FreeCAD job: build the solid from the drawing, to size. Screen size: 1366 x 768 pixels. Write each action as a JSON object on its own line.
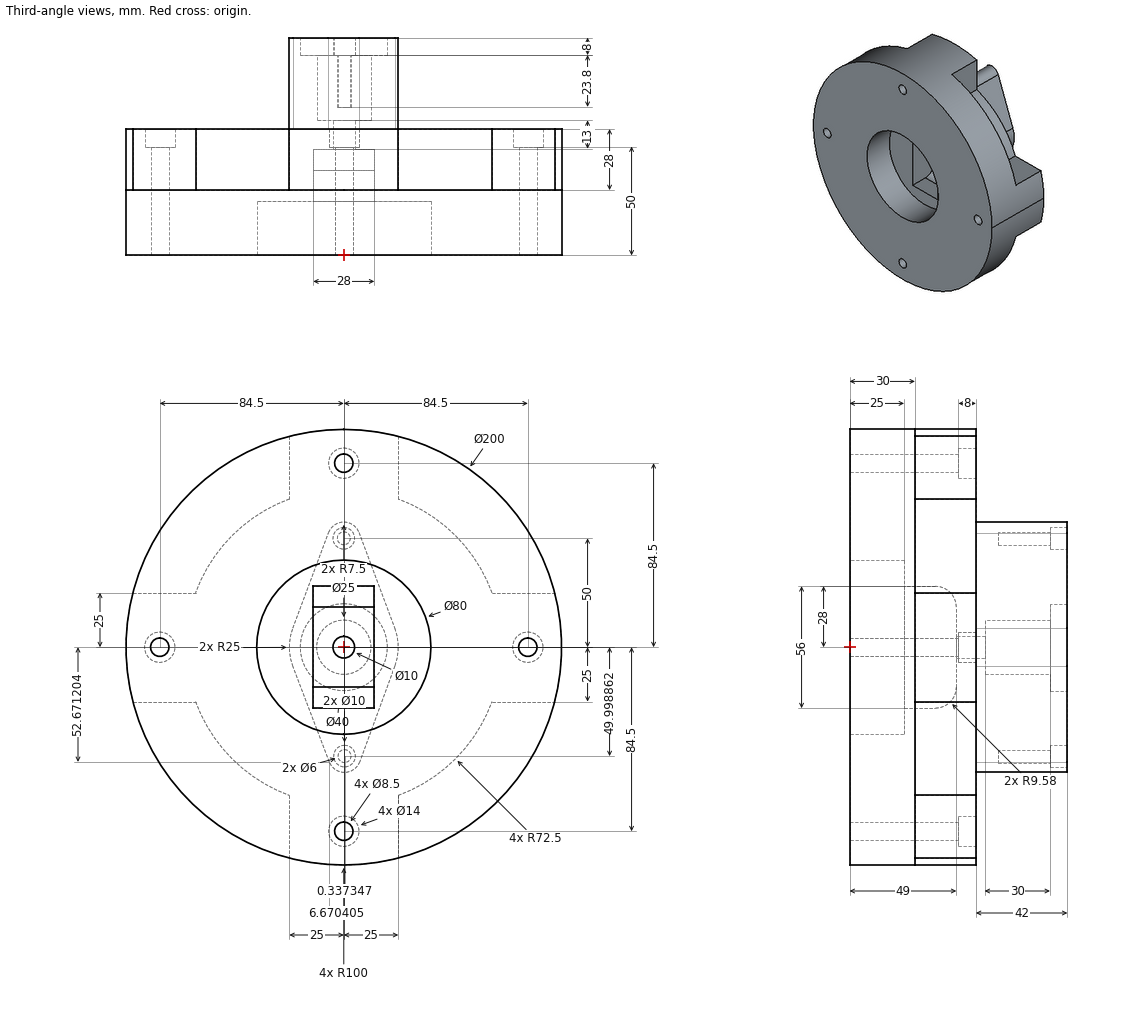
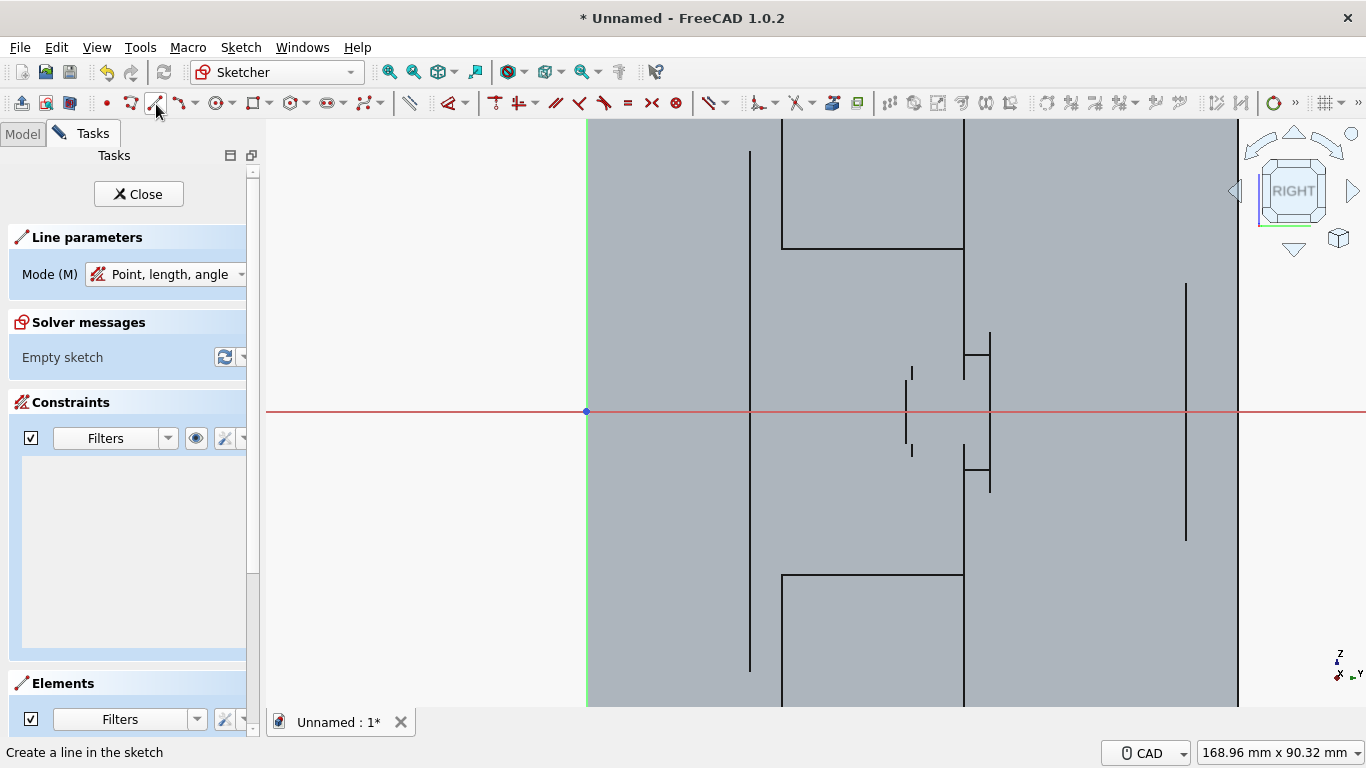
{"action": "left_click", "coordinate": [906, 532]}
{"action": "left_click", "coordinate": [906, 292]}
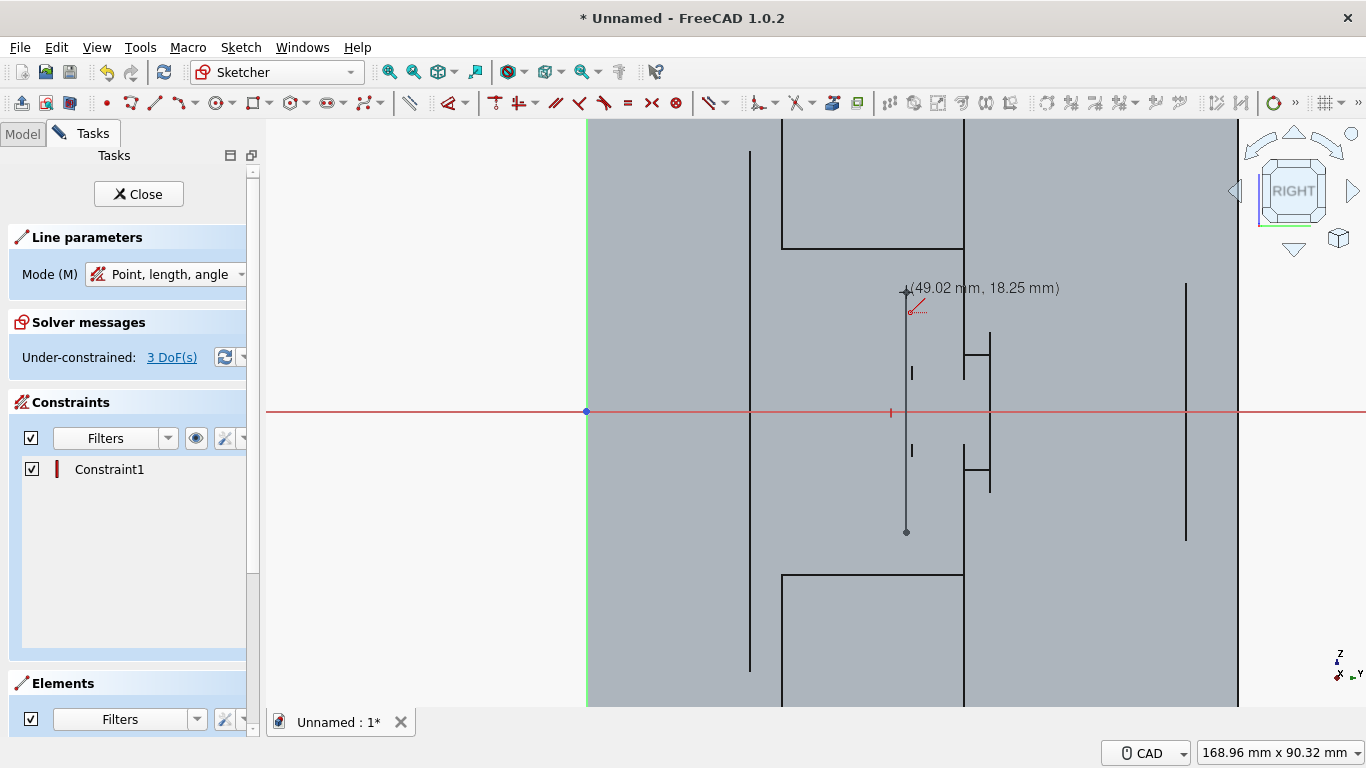
{"action": "key", "text": "g m"}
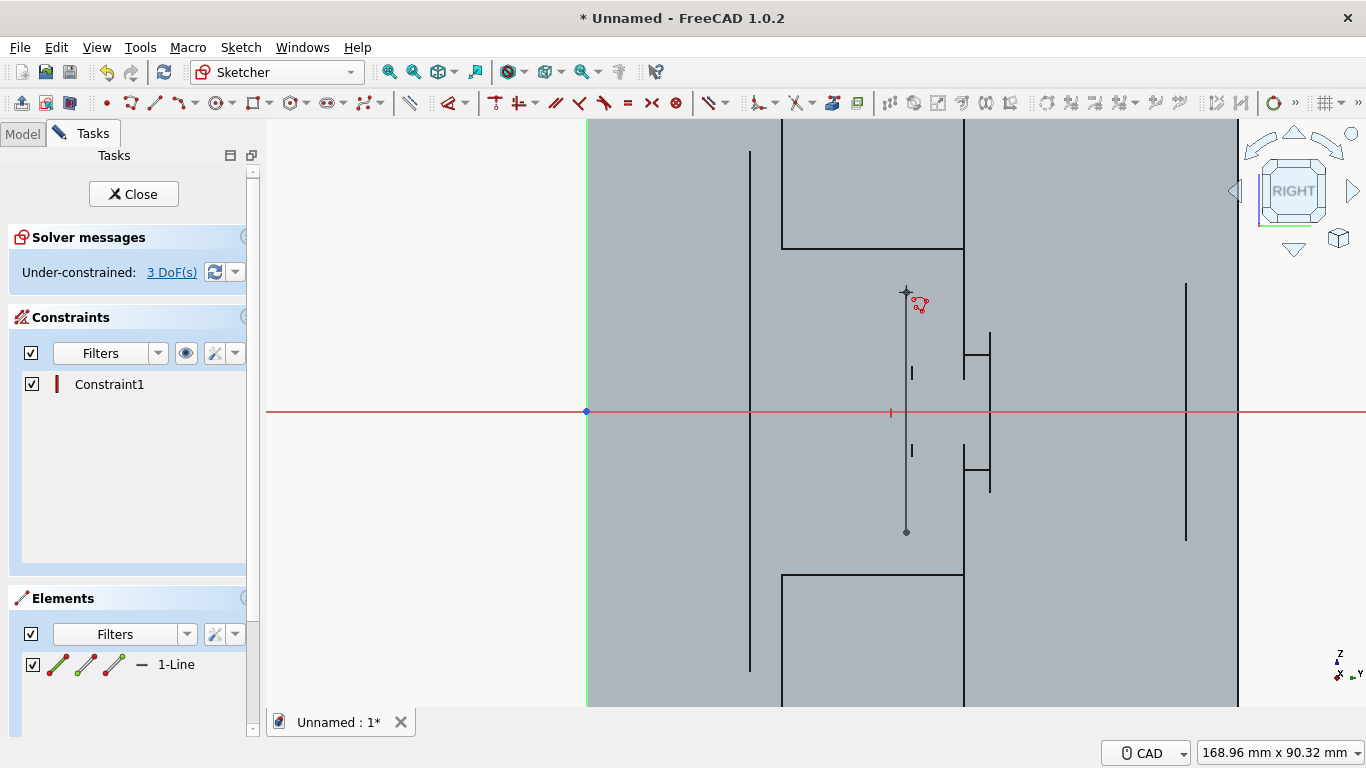
{"action": "left_click", "coordinate": [843, 230]}
{"action": "left_click", "coordinate": [750, 230]}
{"action": "left_click", "coordinate": [750, 594]}
{"action": "left_click", "coordinate": [843, 594]}
{"action": "right_click", "coordinate": [843, 594]}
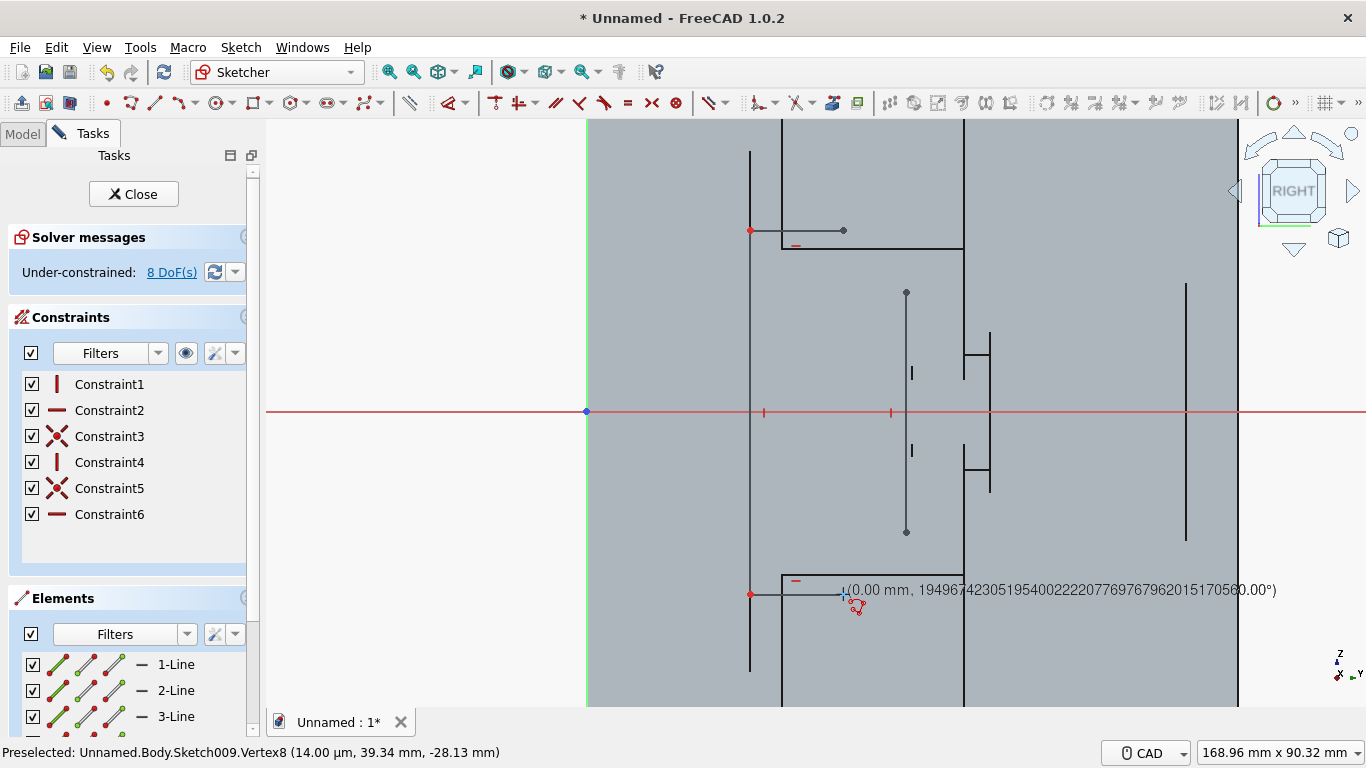
{"action": "key", "text": "g 3 a"}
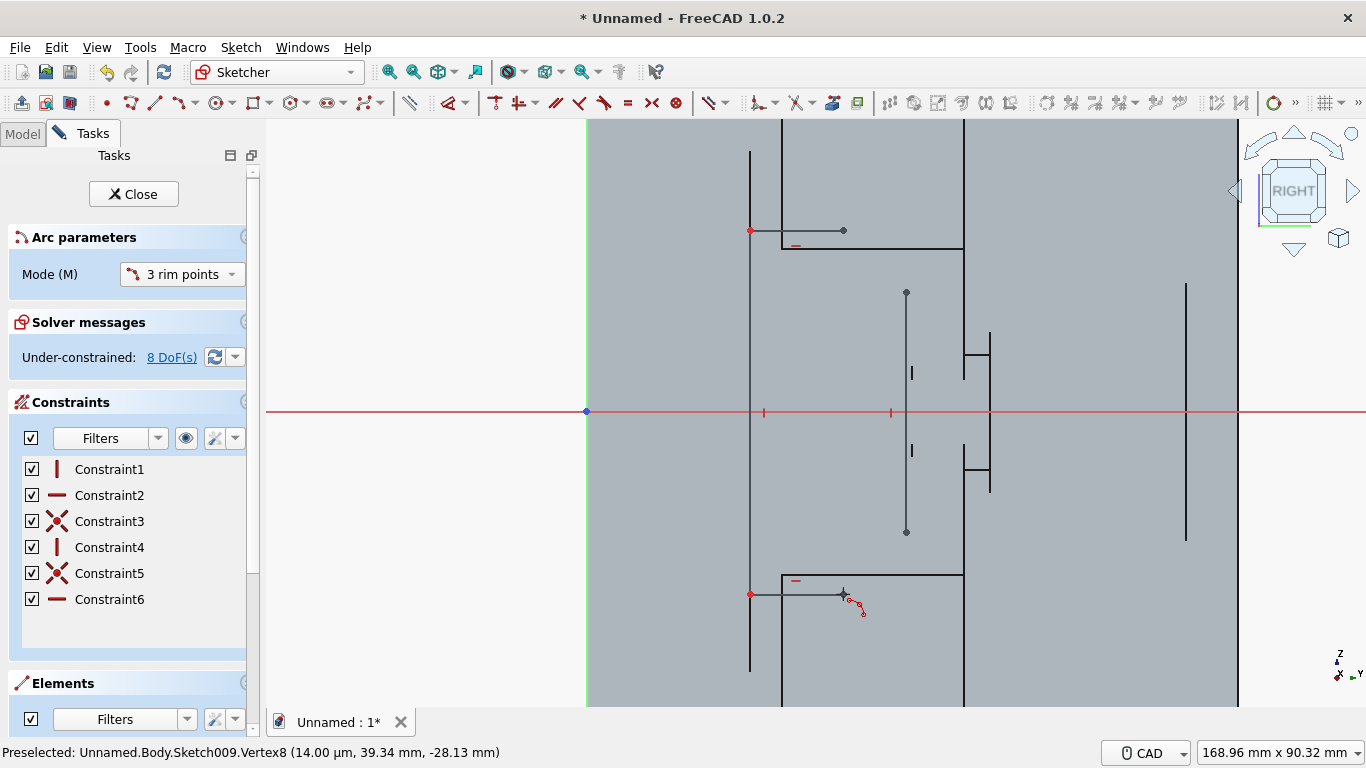
{"action": "left_click", "coordinate": [906, 293]}
{"action": "left_click", "coordinate": [843, 231]}
{"action": "left_click", "coordinate": [888, 248]}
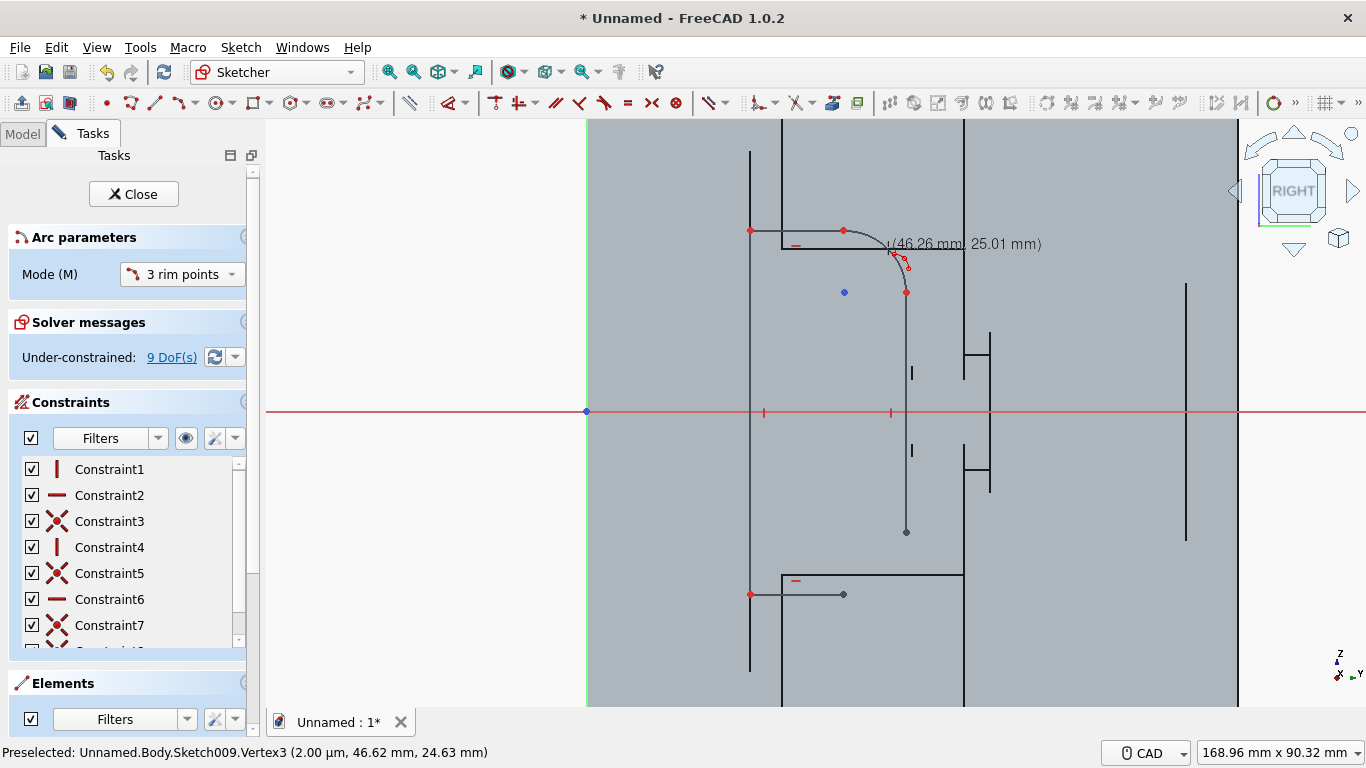
{"action": "left_click", "coordinate": [843, 595]}
{"action": "left_click", "coordinate": [906, 533]}
{"action": "left_click", "coordinate": [888, 576]}
{"action": "key", "text": "Escape"}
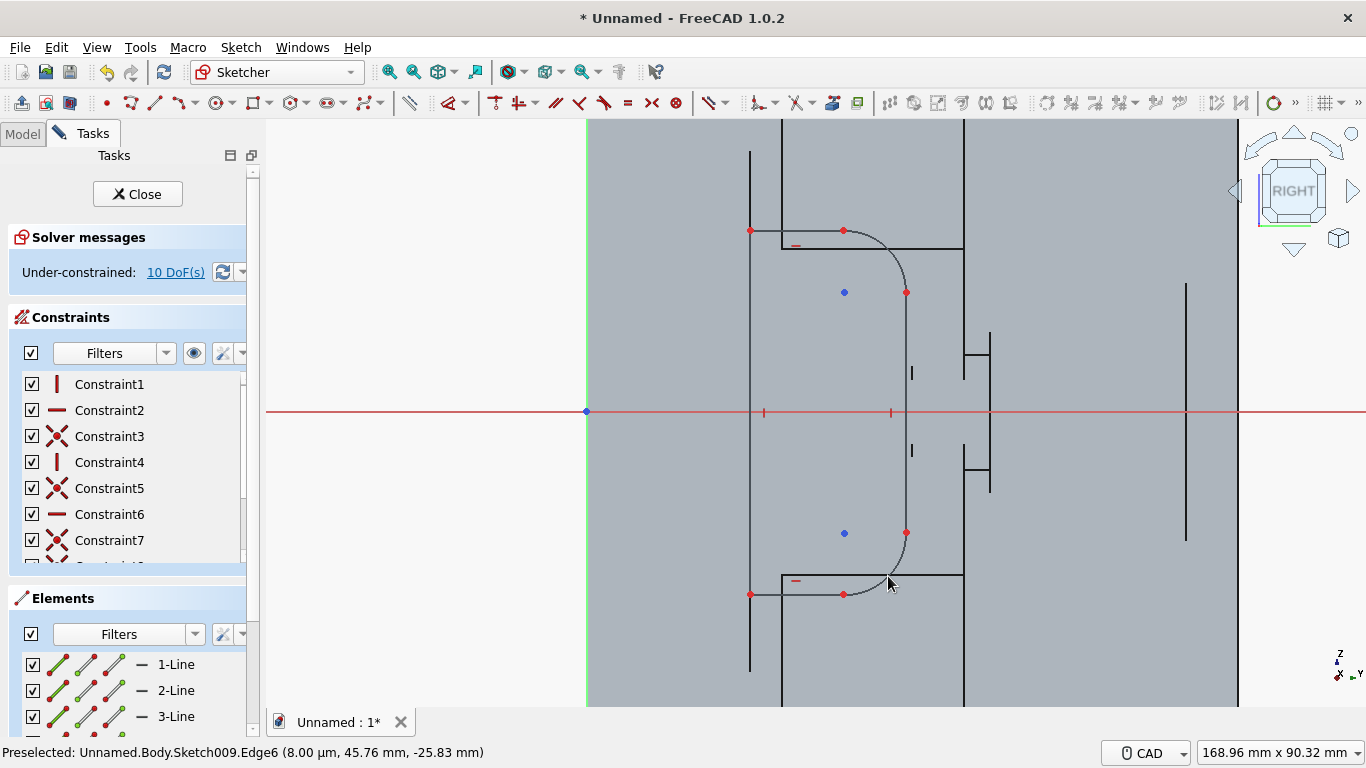
{"action": "left_click", "coordinate": [906, 461]}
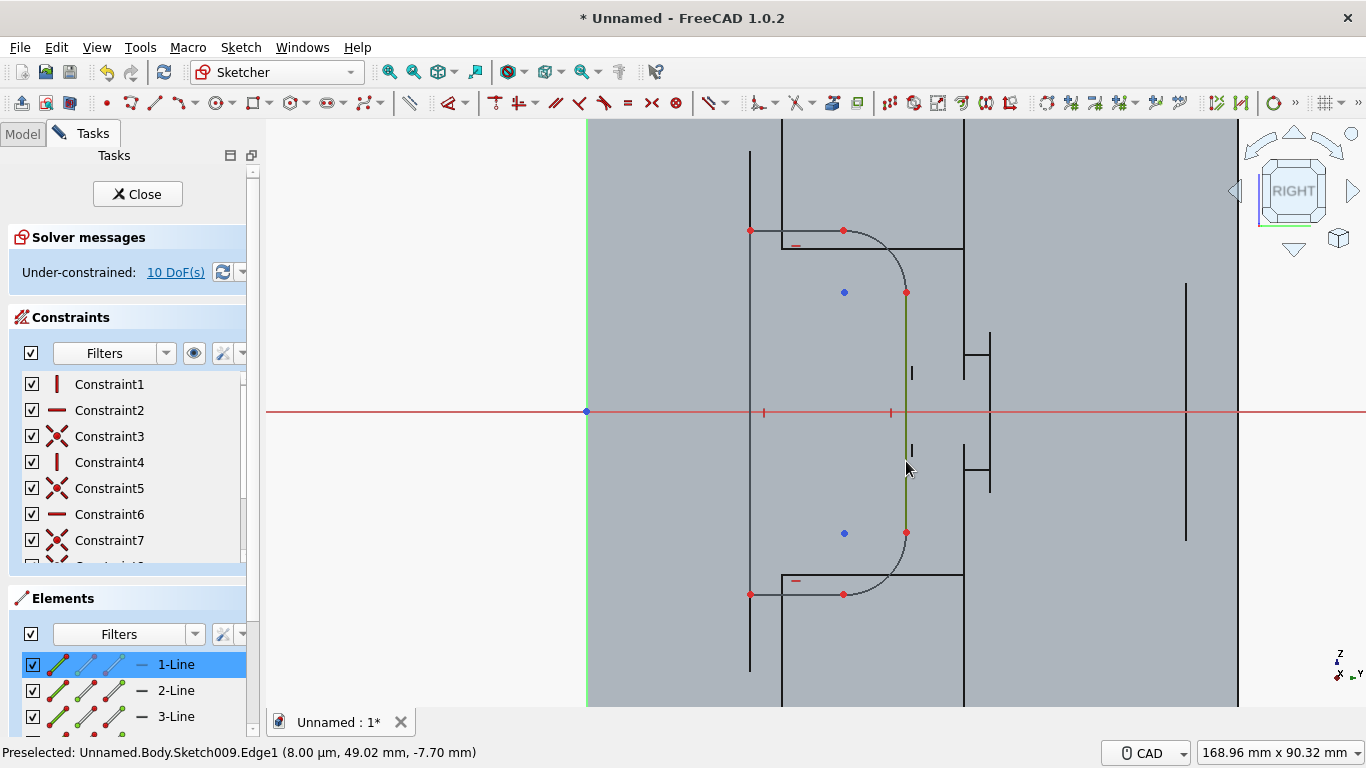
{"action": "left_click", "coordinate": [899, 264]}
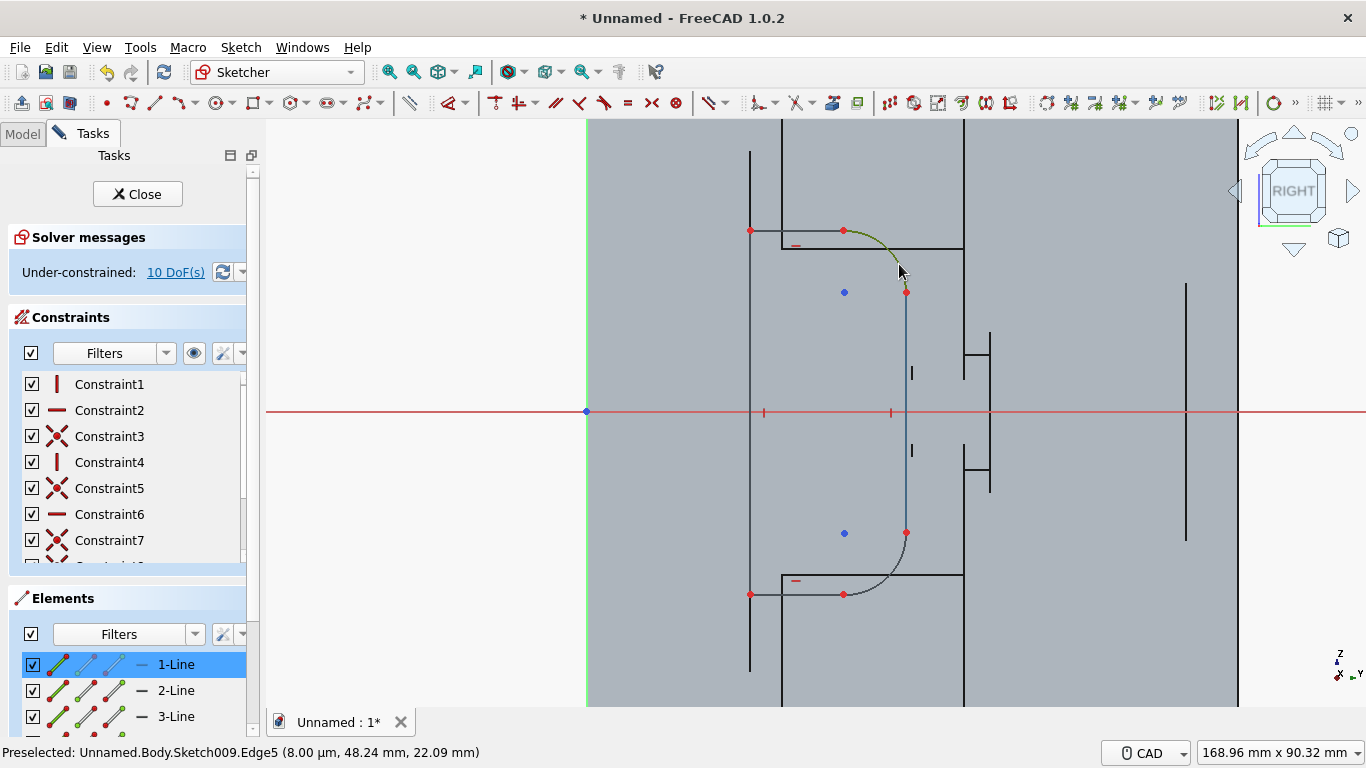
{"action": "key", "text": "t"}